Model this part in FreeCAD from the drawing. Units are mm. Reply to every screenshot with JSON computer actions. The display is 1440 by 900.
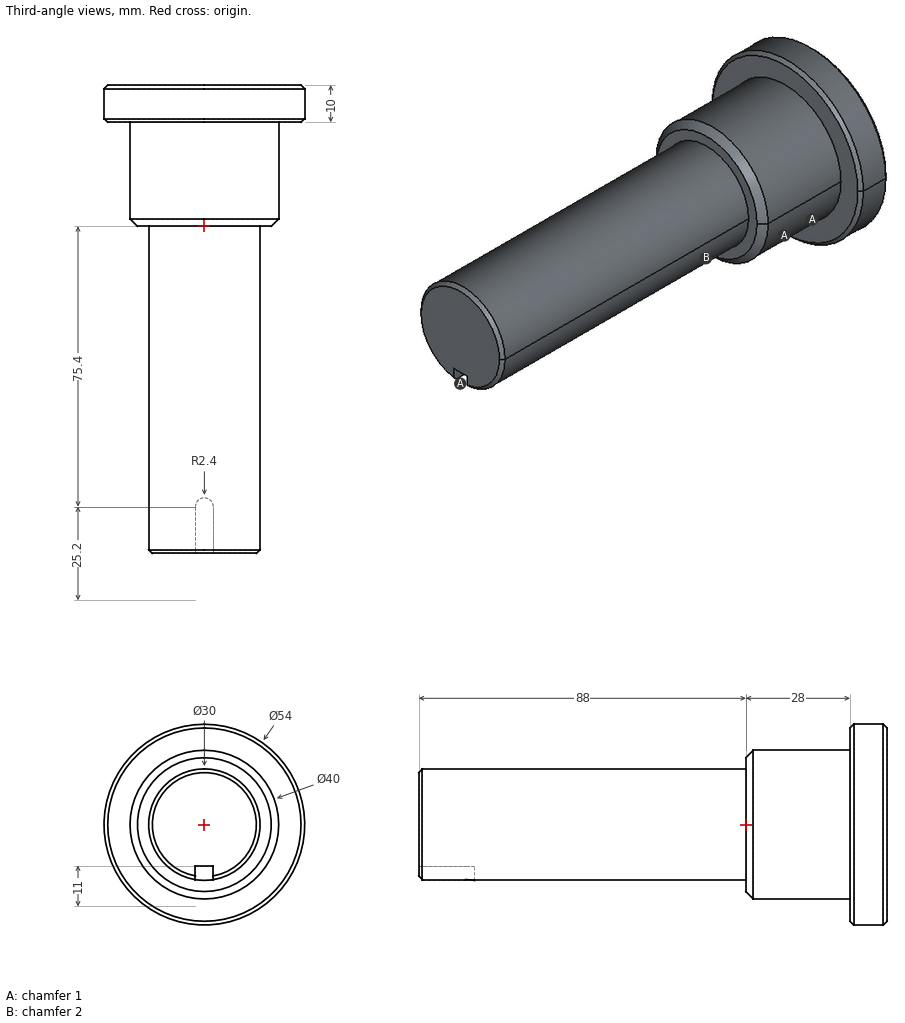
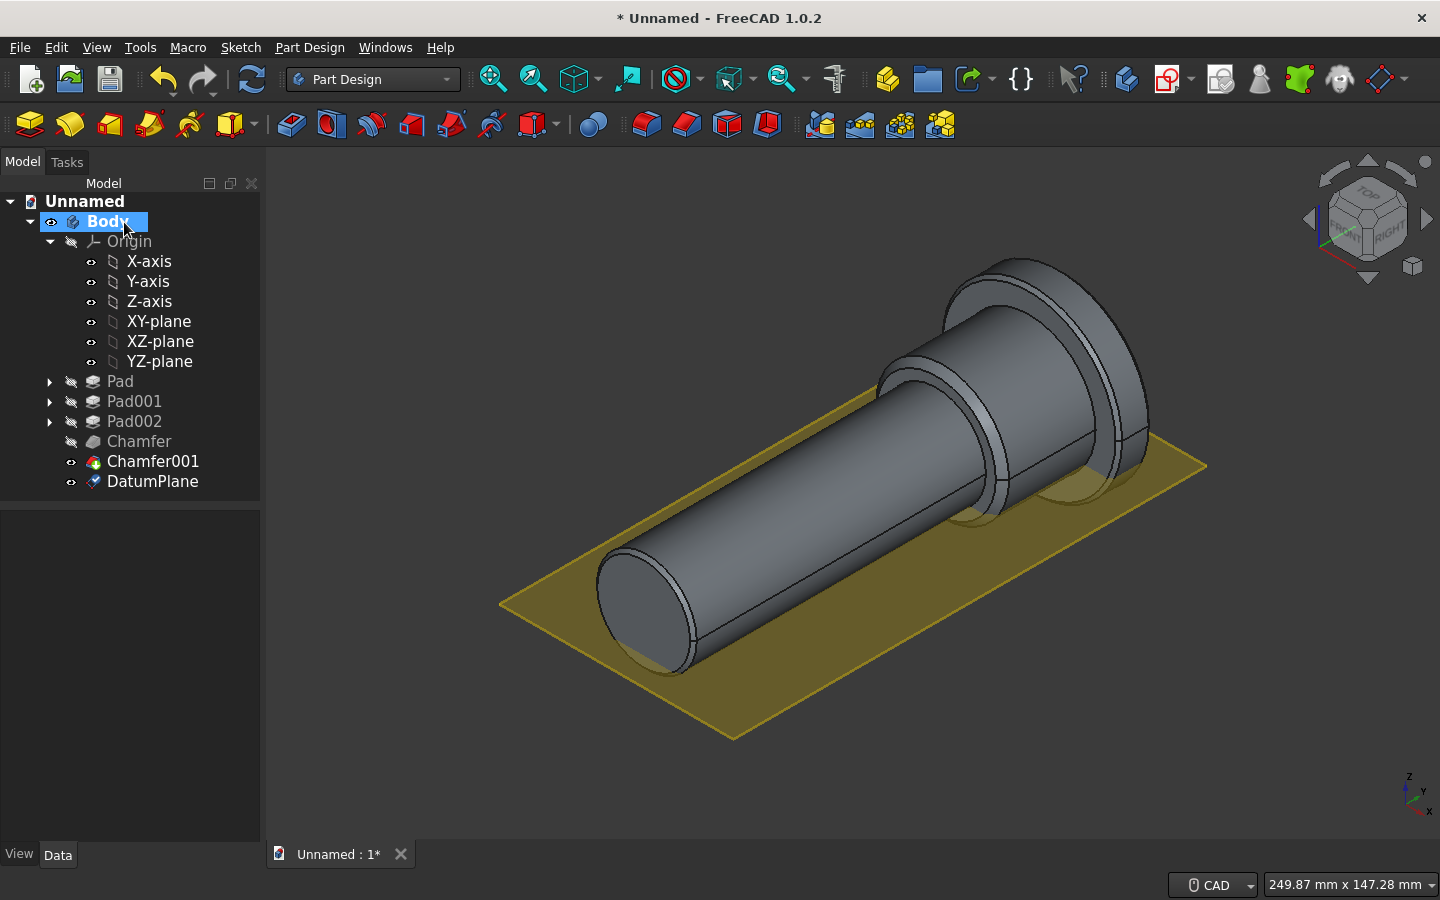
{"action": "left_click", "coordinate": [116, 482]}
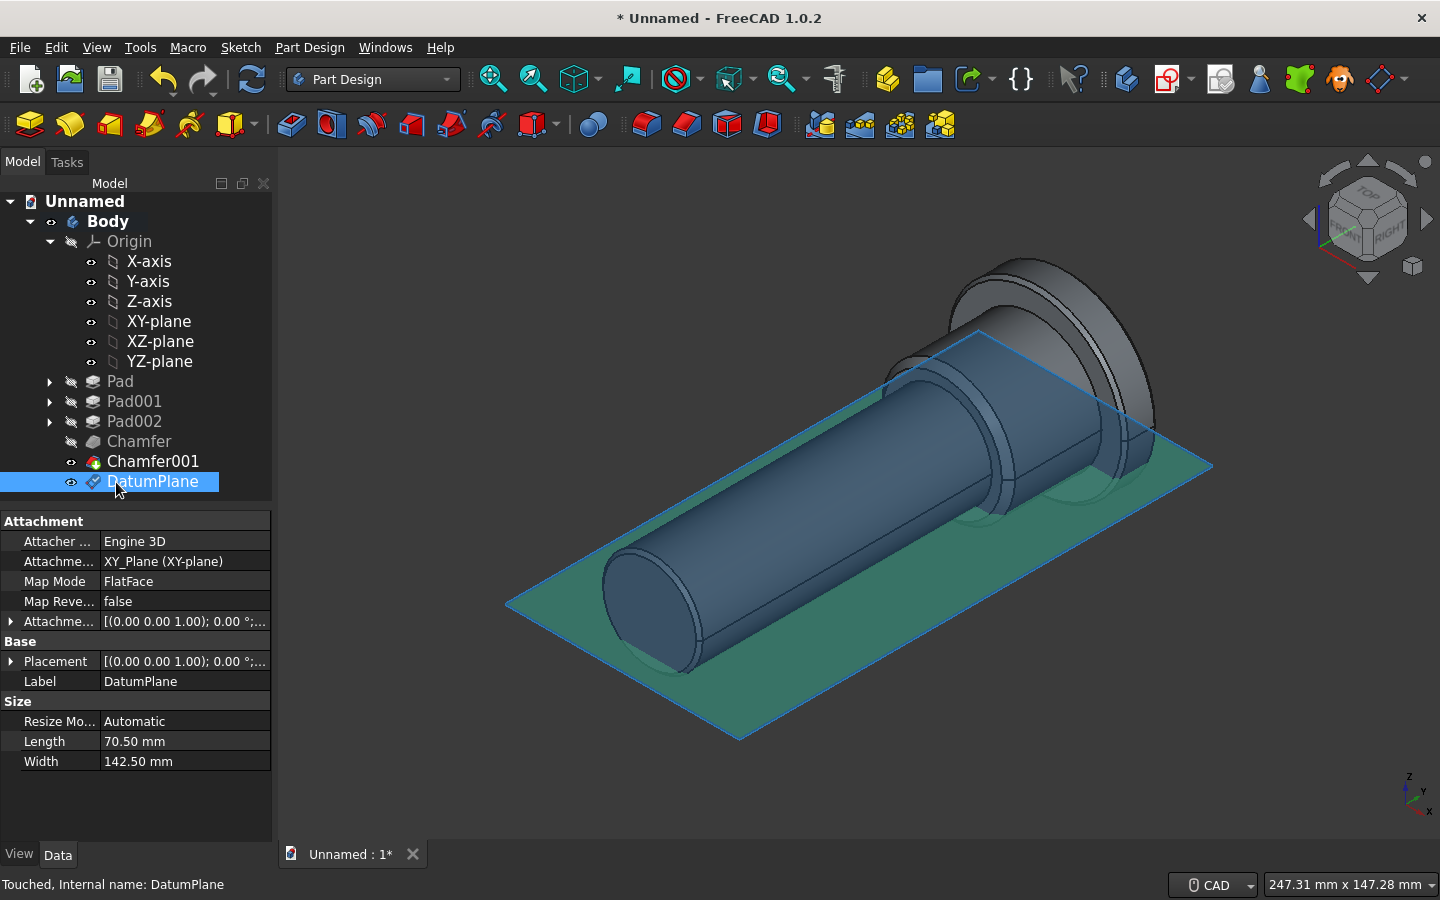
{"action": "left_click", "coordinate": [1168, 80]}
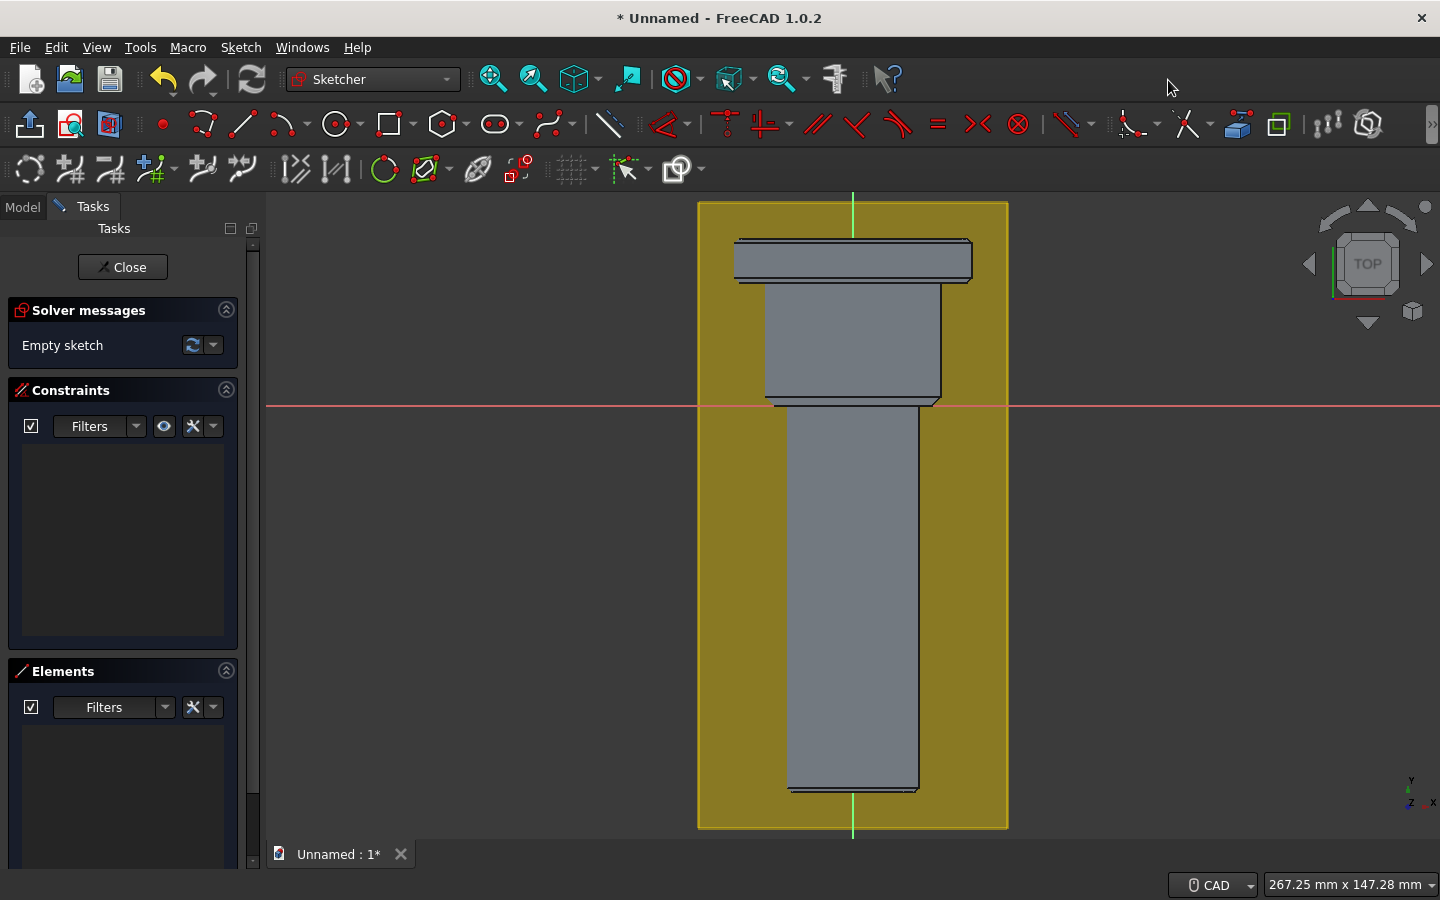
{"action": "key", "text": "q s"}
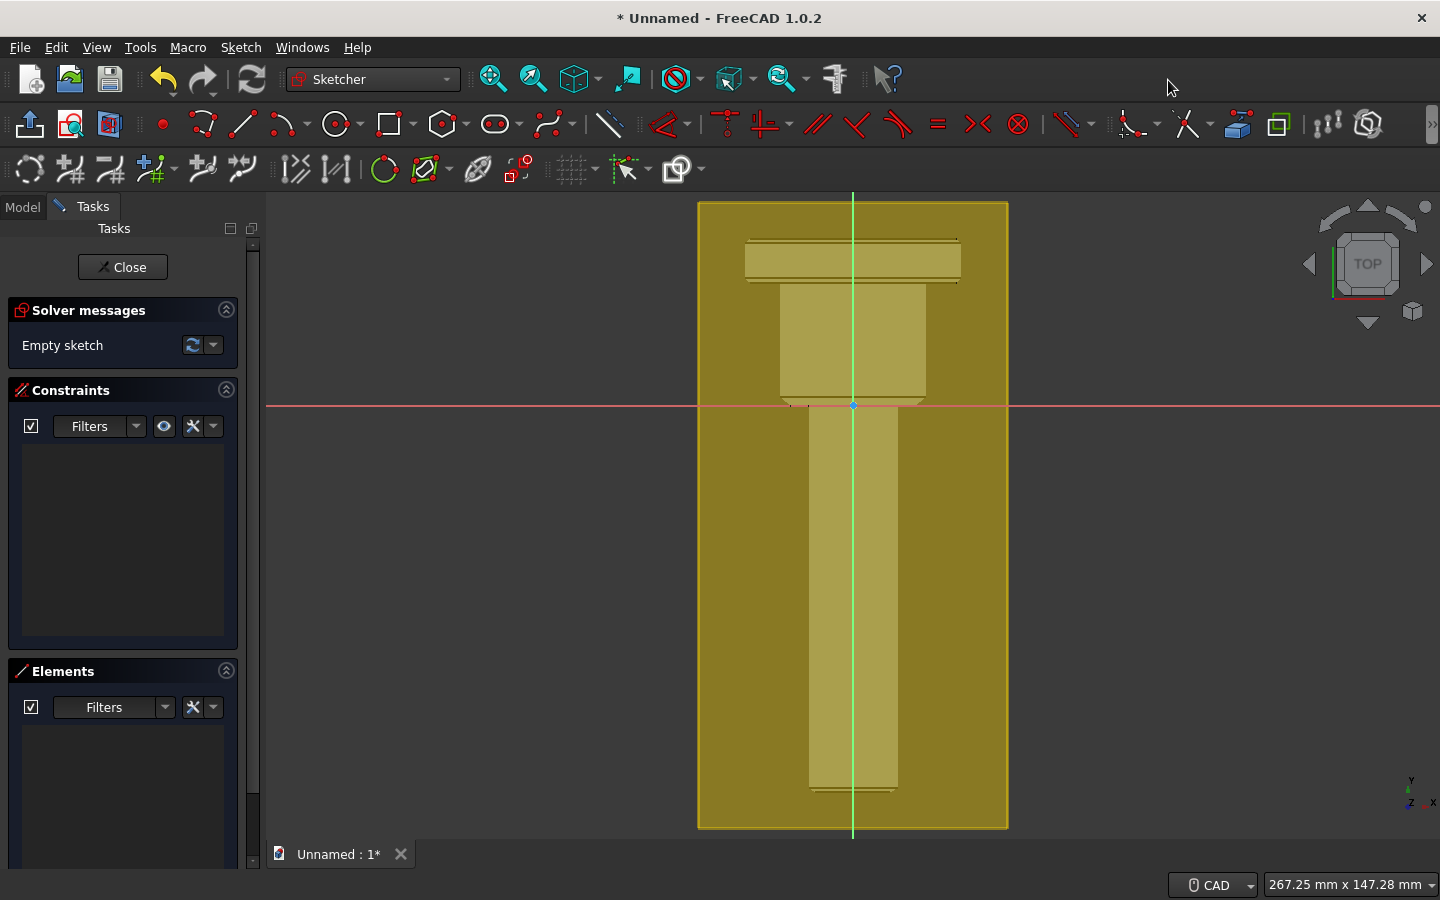
{"action": "scroll", "coordinate": [784, 516], "scroll_direction": "down", "scroll_amount": 5}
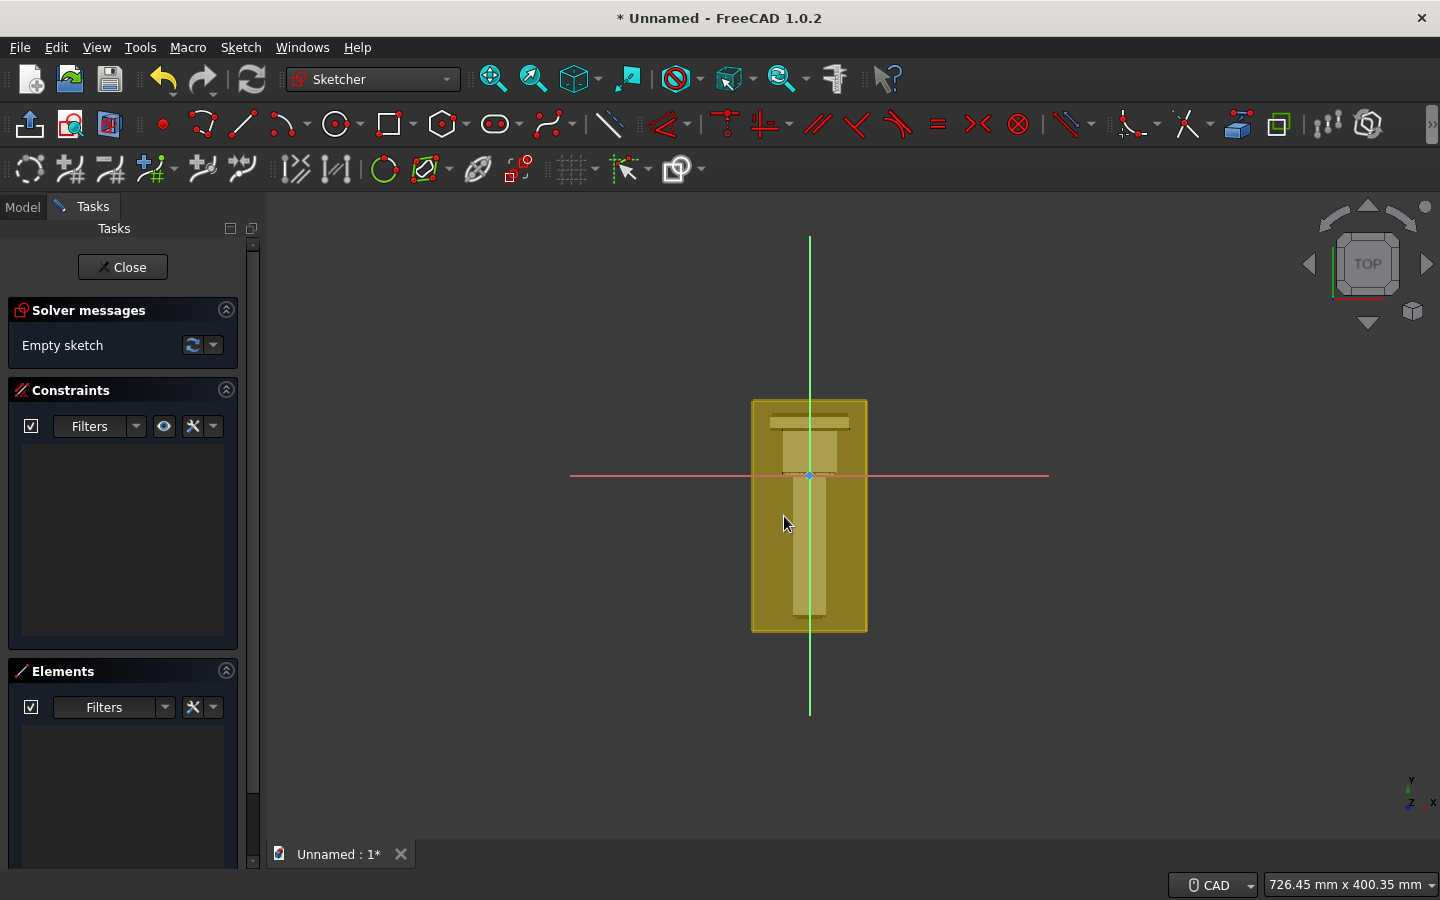
{"action": "scroll", "coordinate": [813, 629], "scroll_direction": "up", "scroll_amount": 11}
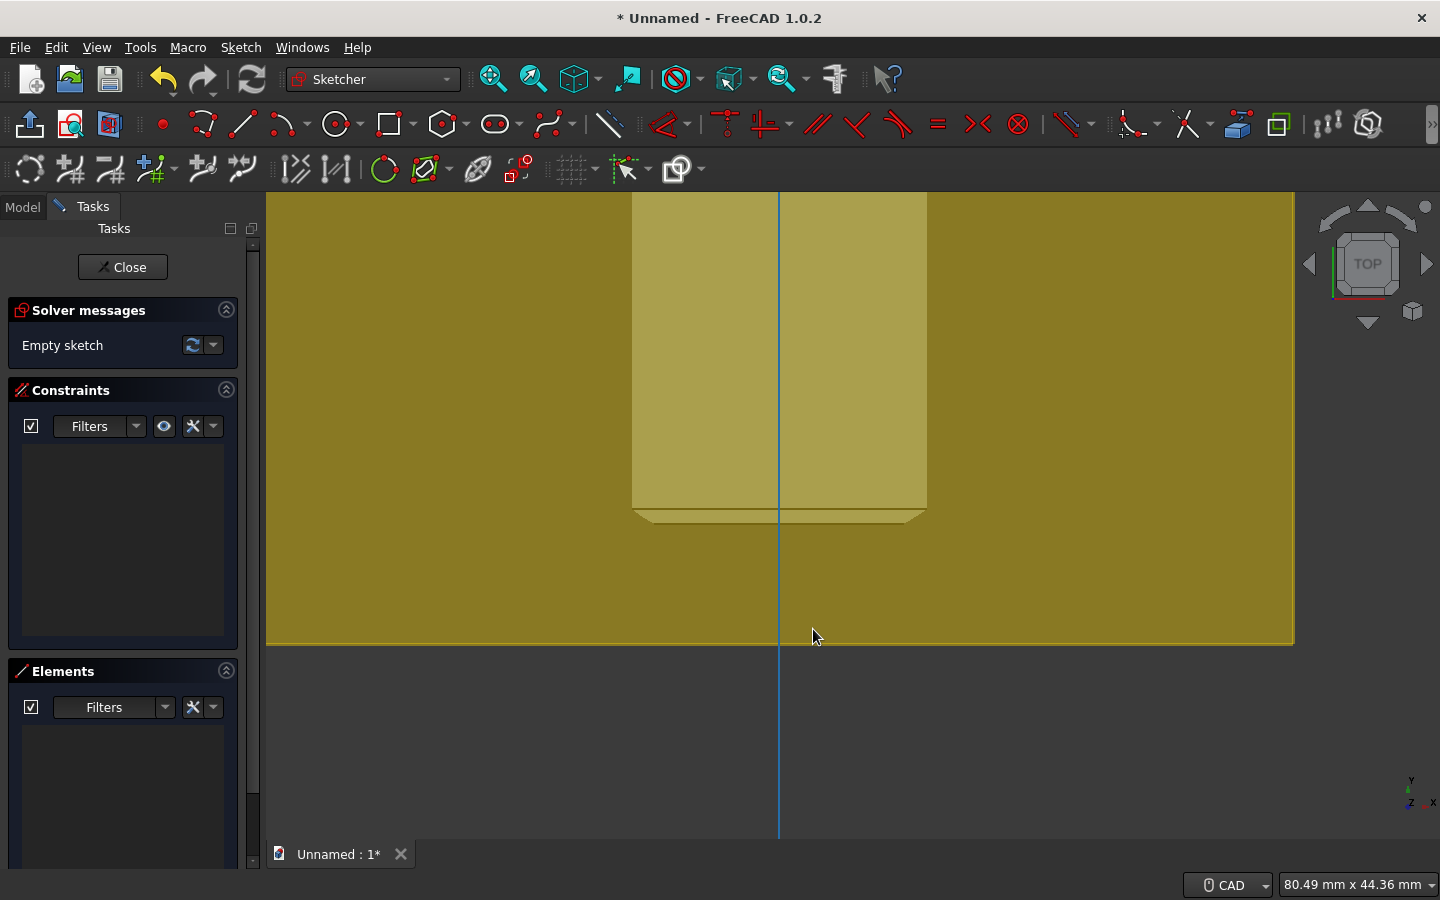
{"action": "left_click", "coordinate": [204, 124]}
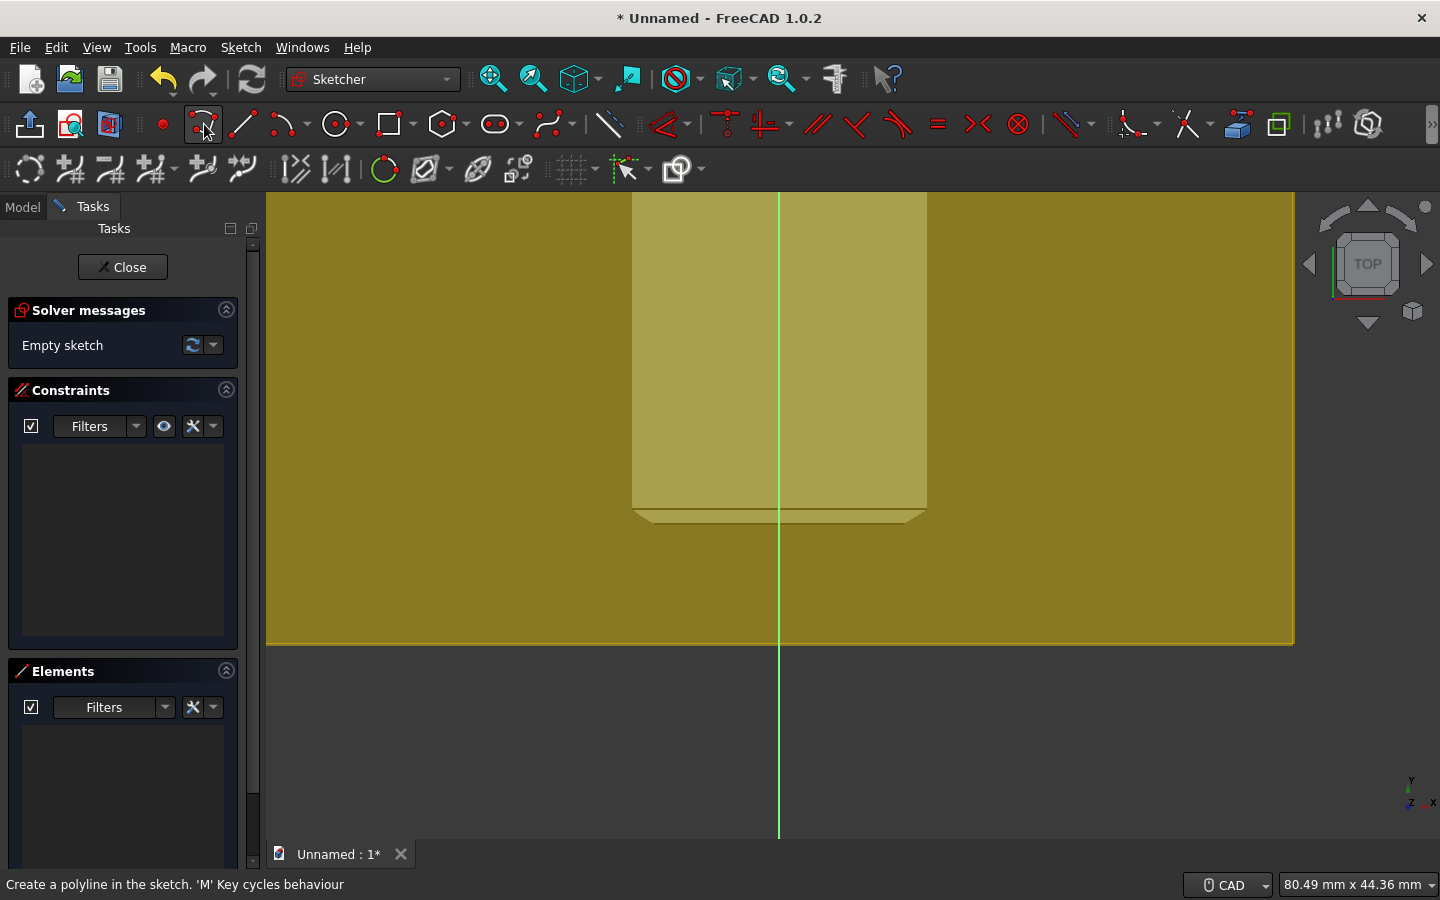
{"action": "left_click", "coordinate": [744, 340]}
{"action": "left_click", "coordinate": [744, 708]}
{"action": "left_click", "coordinate": [814, 708]}
{"action": "left_click", "coordinate": [814, 340]}
{"action": "right_click", "coordinate": [814, 340]}